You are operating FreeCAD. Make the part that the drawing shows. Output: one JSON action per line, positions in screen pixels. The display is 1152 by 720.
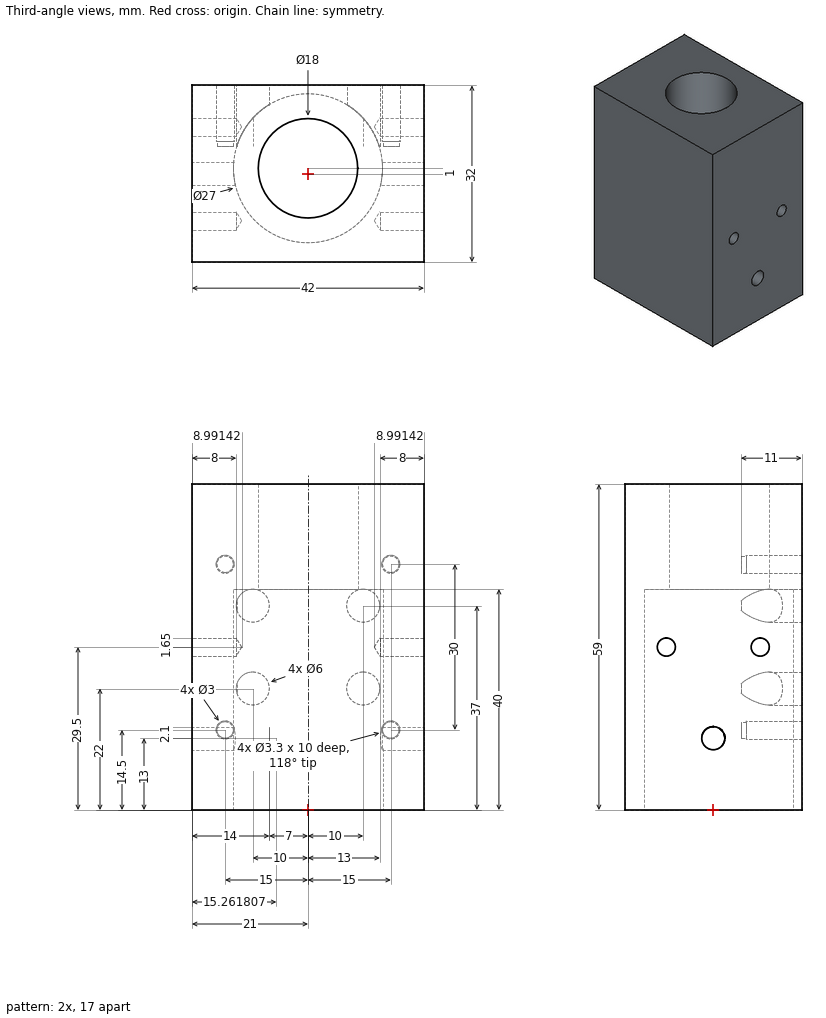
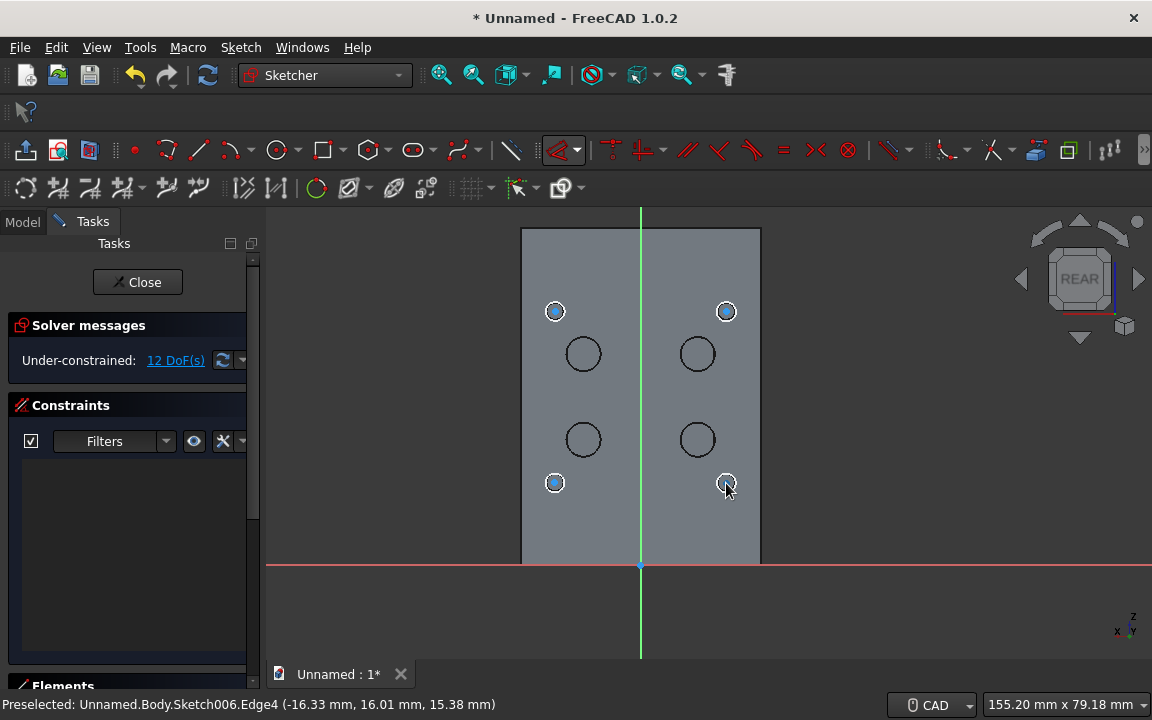
{"action": "scroll", "coordinate": [562, 476], "scroll_direction": "up", "scroll_amount": 2}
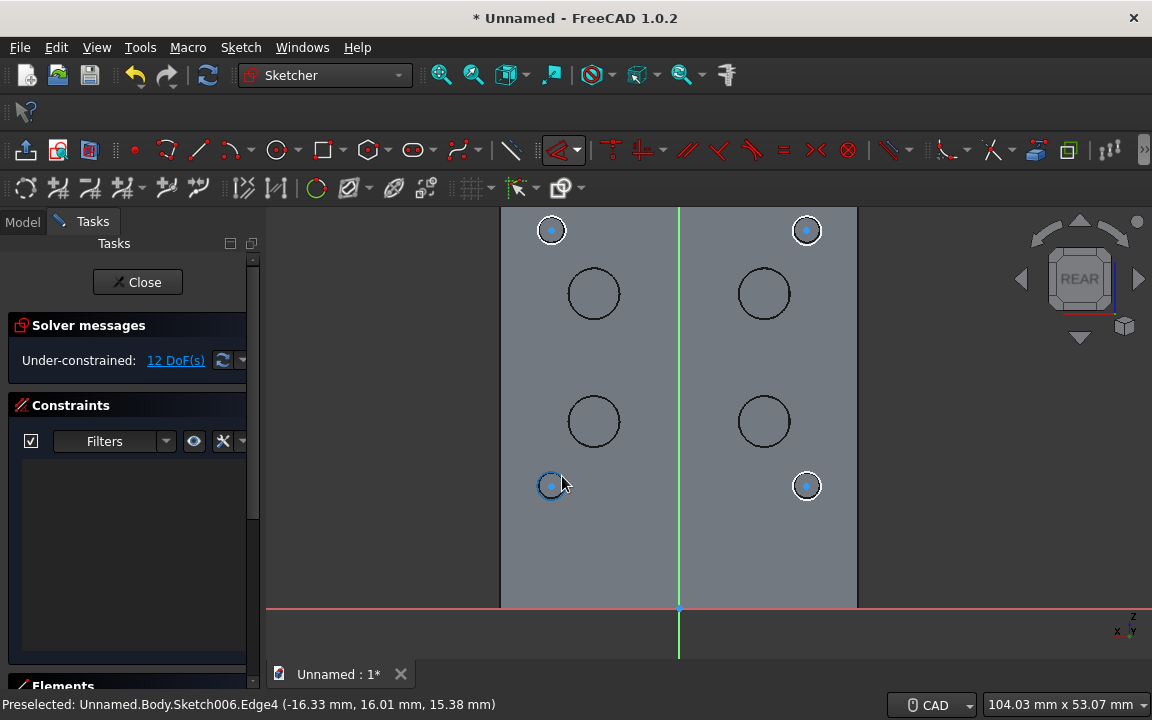
{"action": "left_click", "coordinate": [561, 476]}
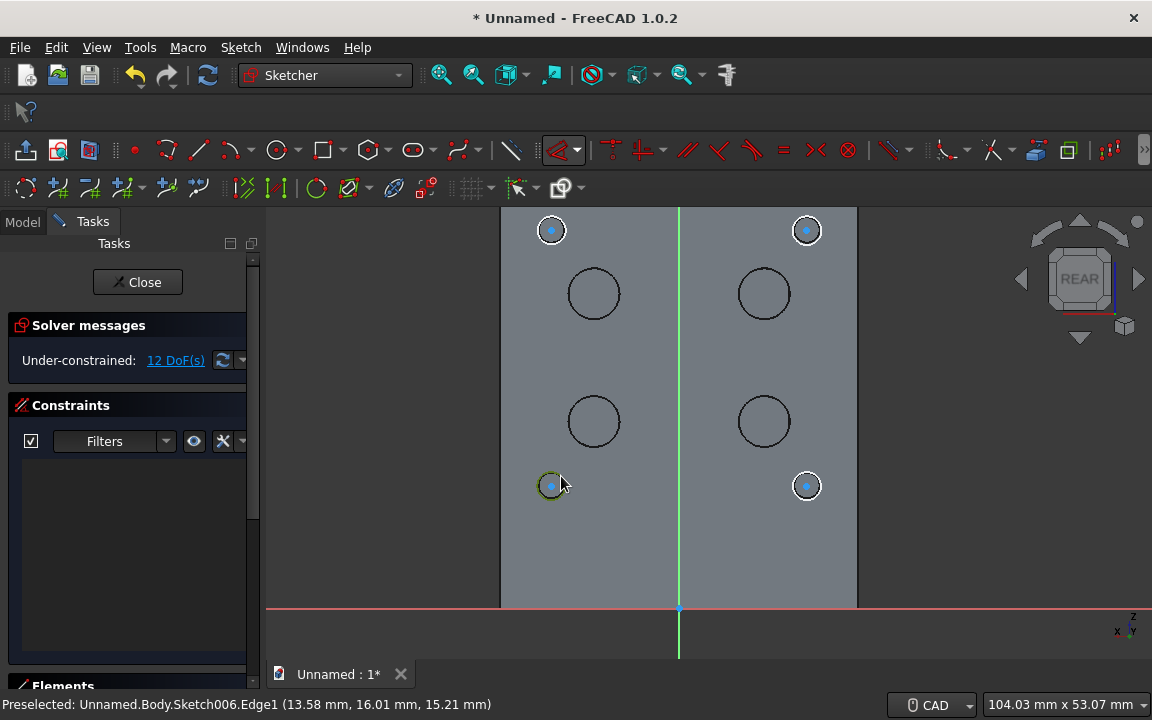
{"action": "left_click", "coordinate": [542, 240]}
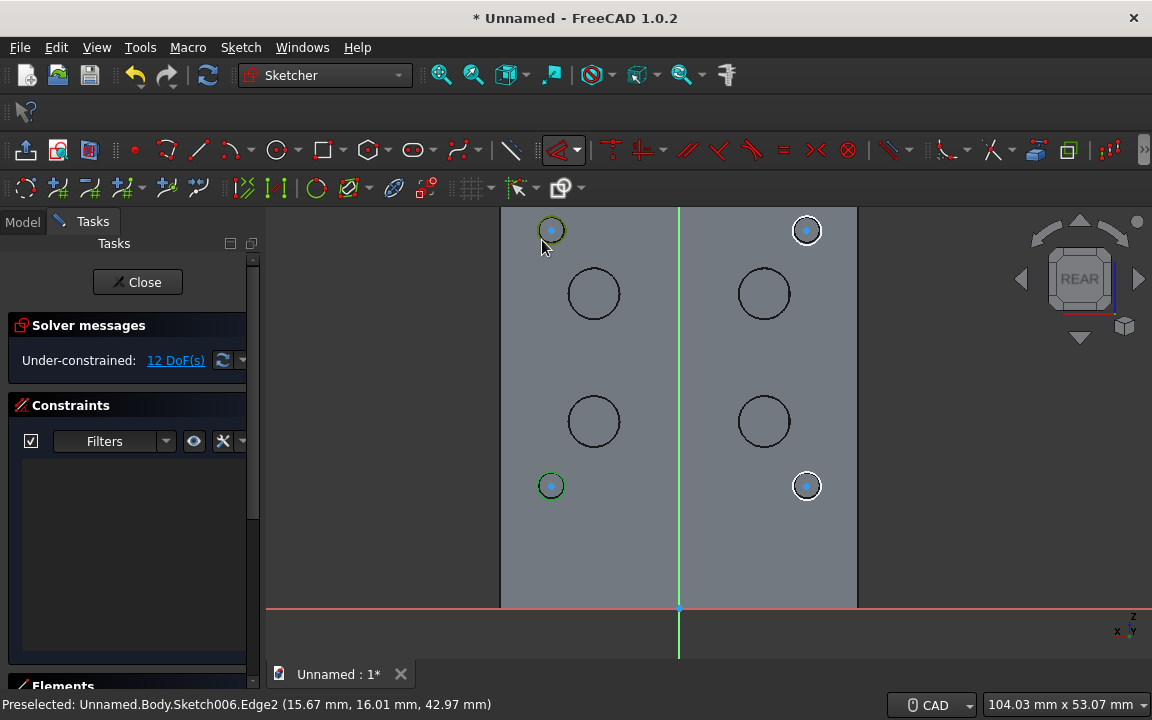
{"action": "left_click", "coordinate": [797, 241]}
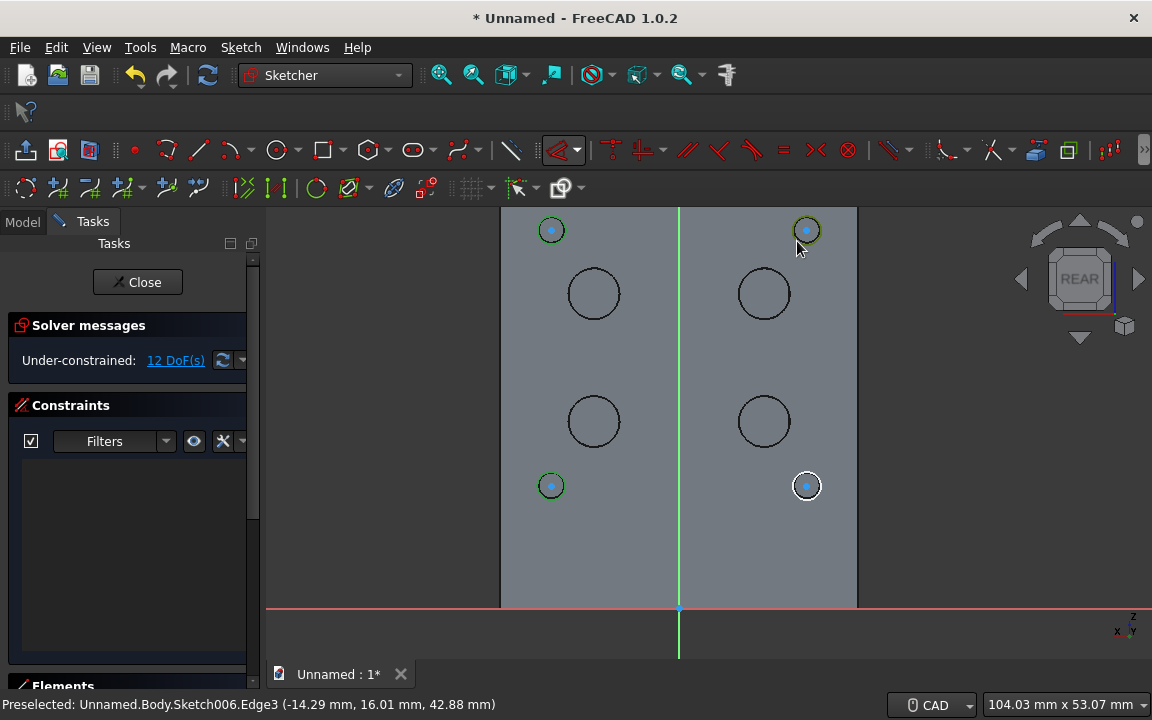
{"action": "left_click", "coordinate": [817, 476]}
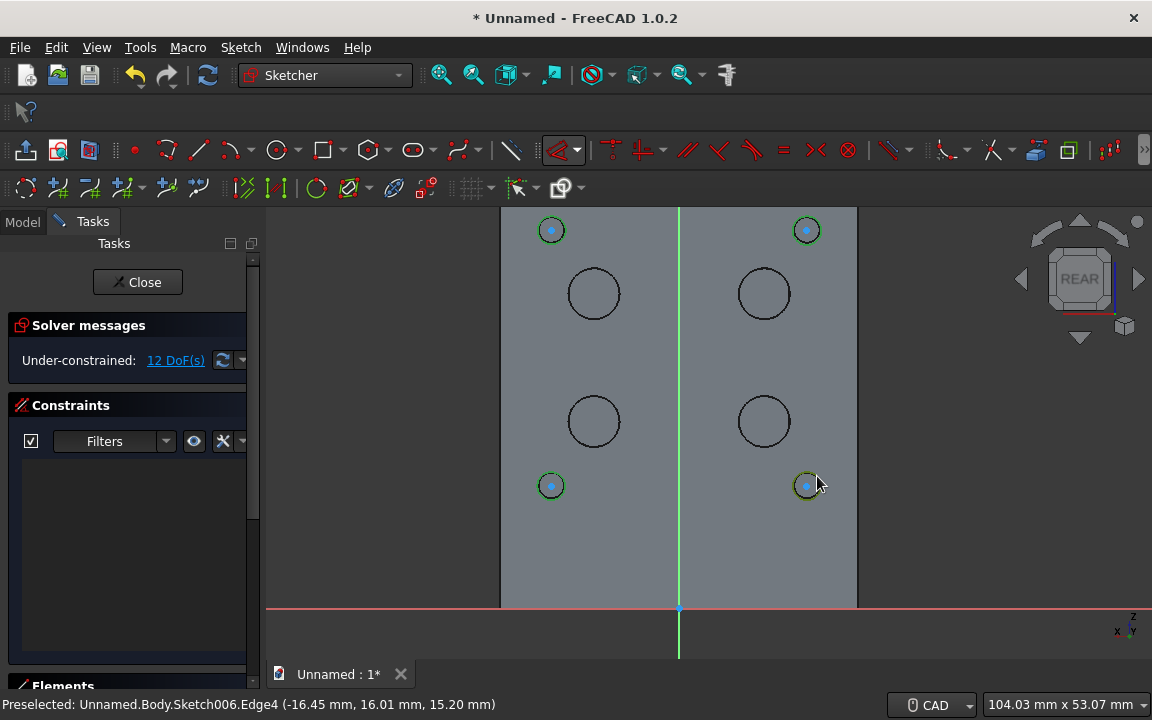
{"action": "key", "text": "e"}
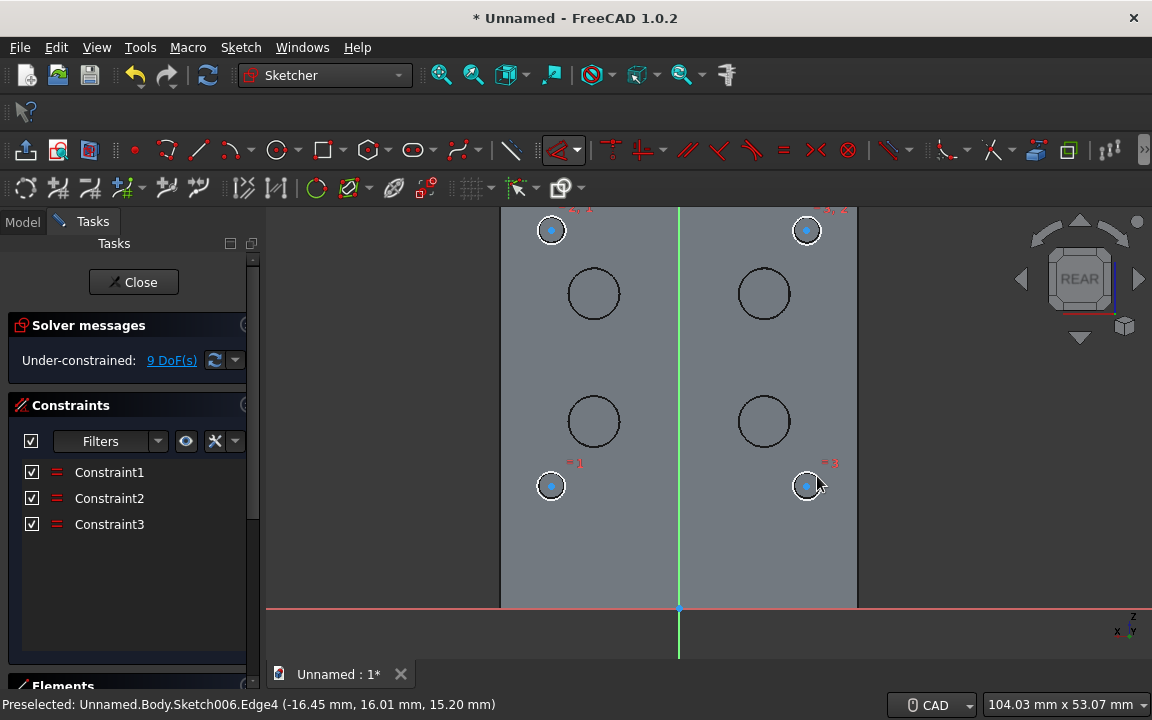
{"action": "scroll", "coordinate": [562, 475], "scroll_direction": "down", "scroll_amount": 2}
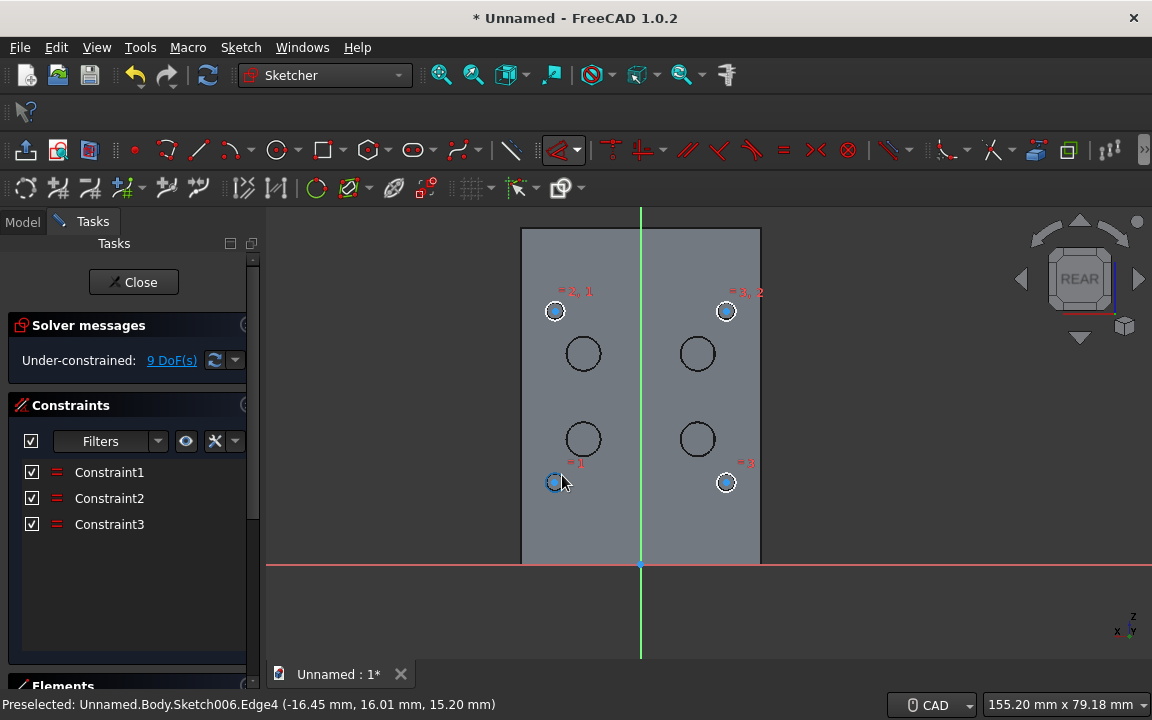
{"action": "left_click", "coordinate": [555, 311]}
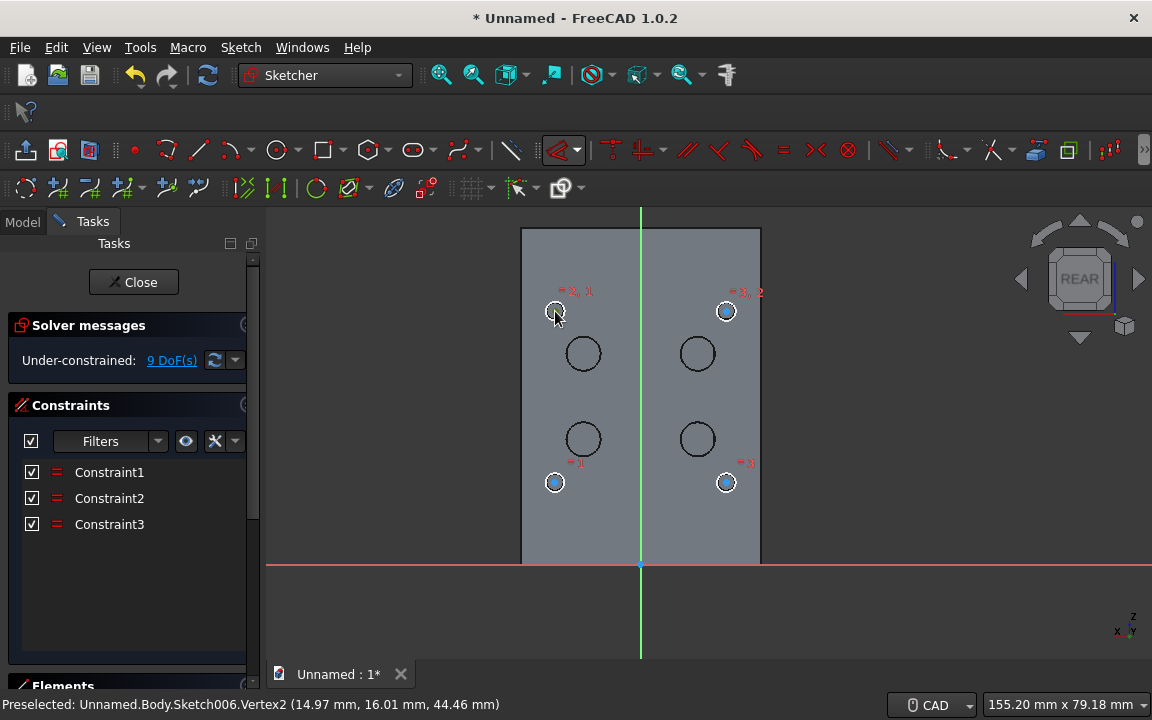
{"action": "left_click", "coordinate": [726, 311]}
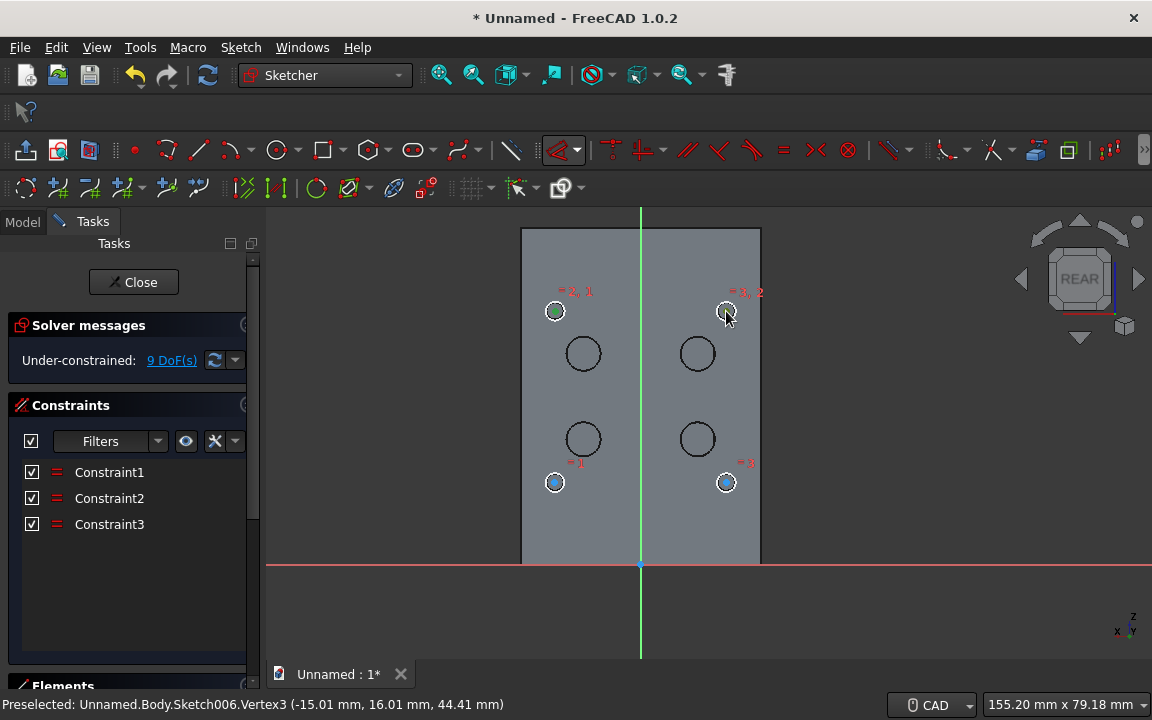
{"action": "left_click", "coordinate": [641, 603]}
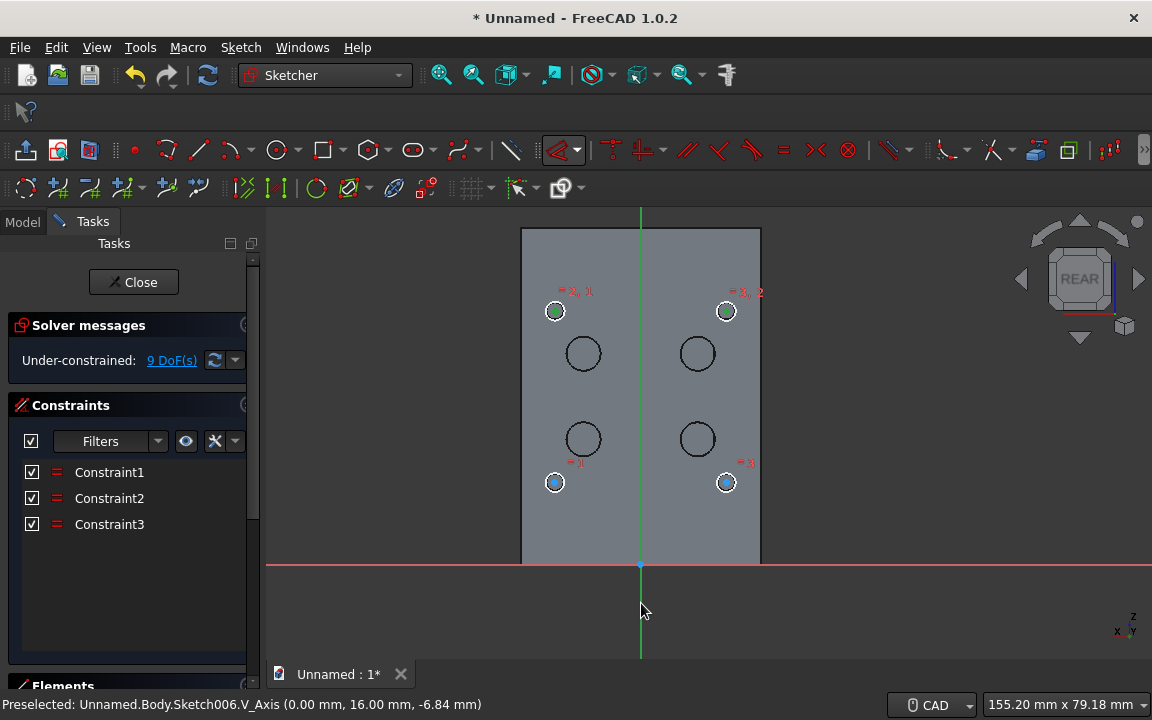
{"action": "key", "text": "s"}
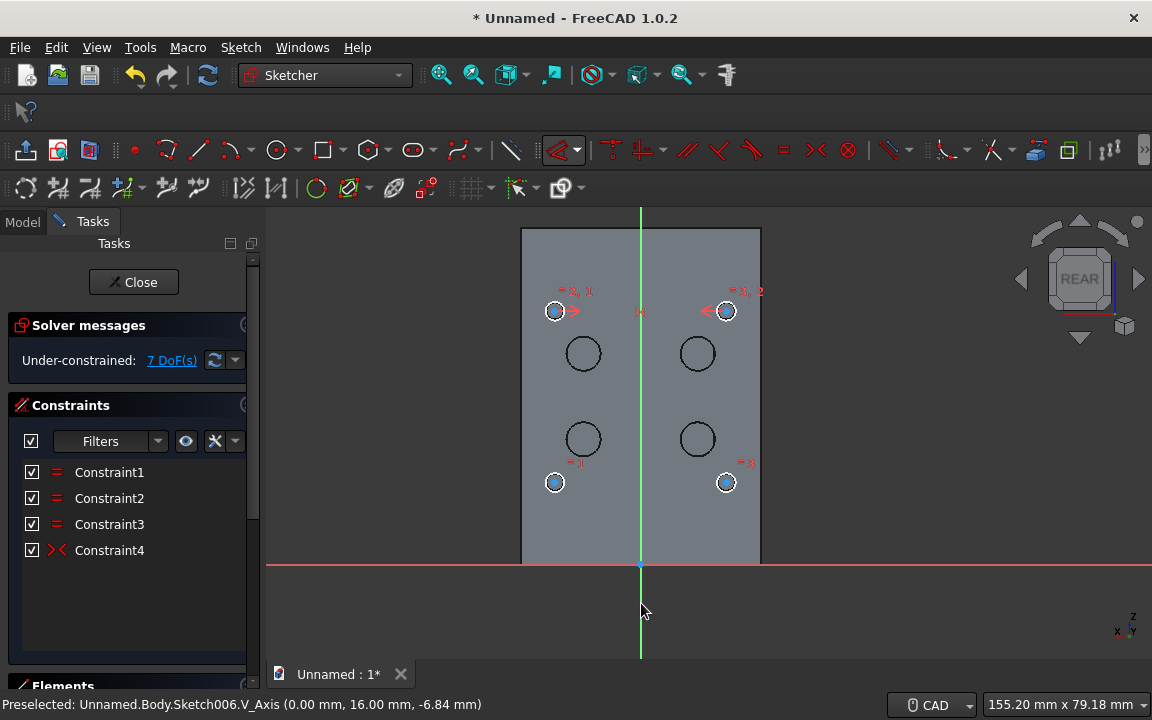
{"action": "left_click", "coordinate": [555, 483]}